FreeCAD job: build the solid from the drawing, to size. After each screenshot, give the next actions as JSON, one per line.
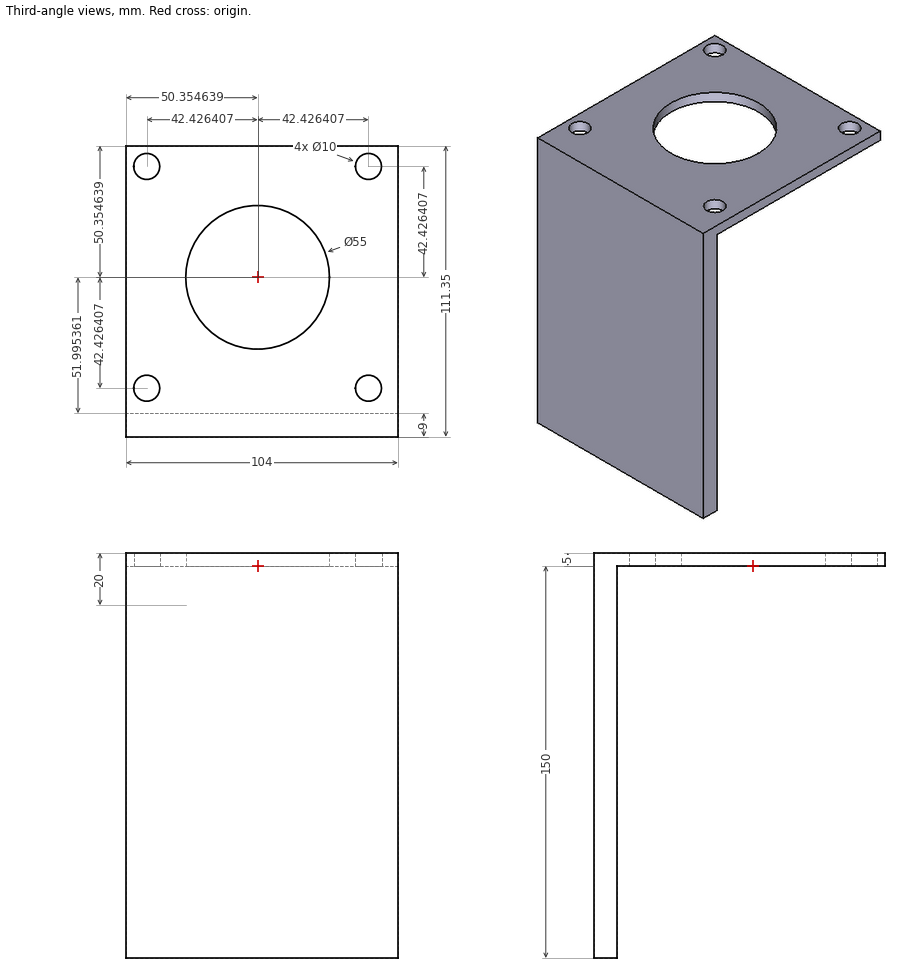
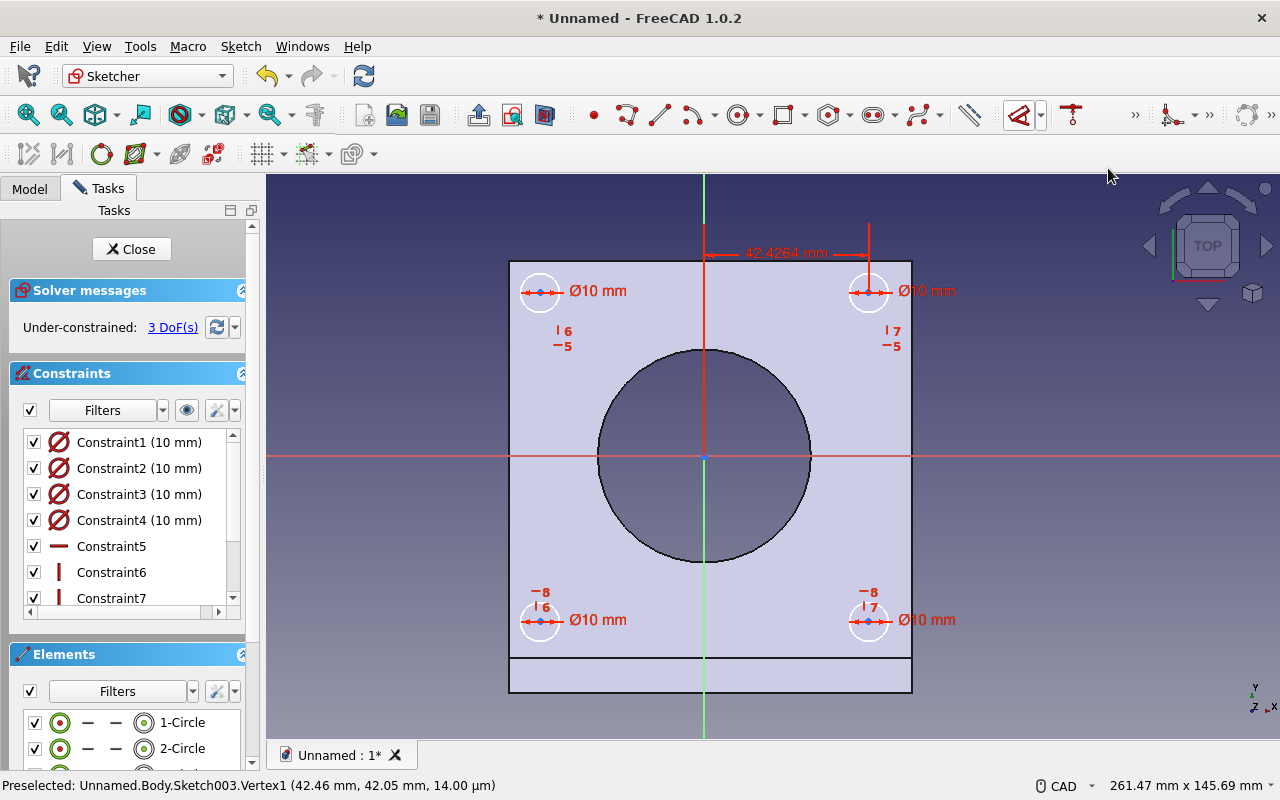
{"action": "left_click", "coordinate": [869, 293]}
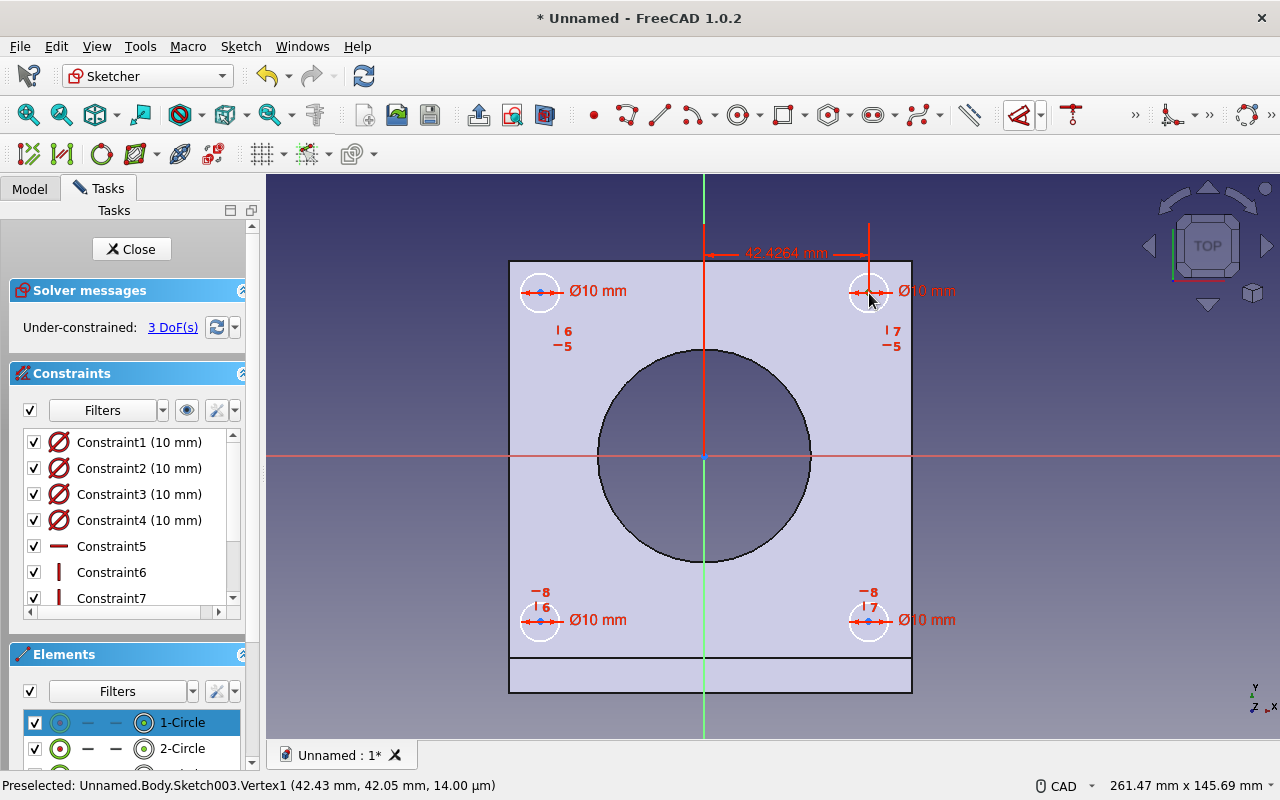
{"action": "left_click", "coordinate": [1040, 116]}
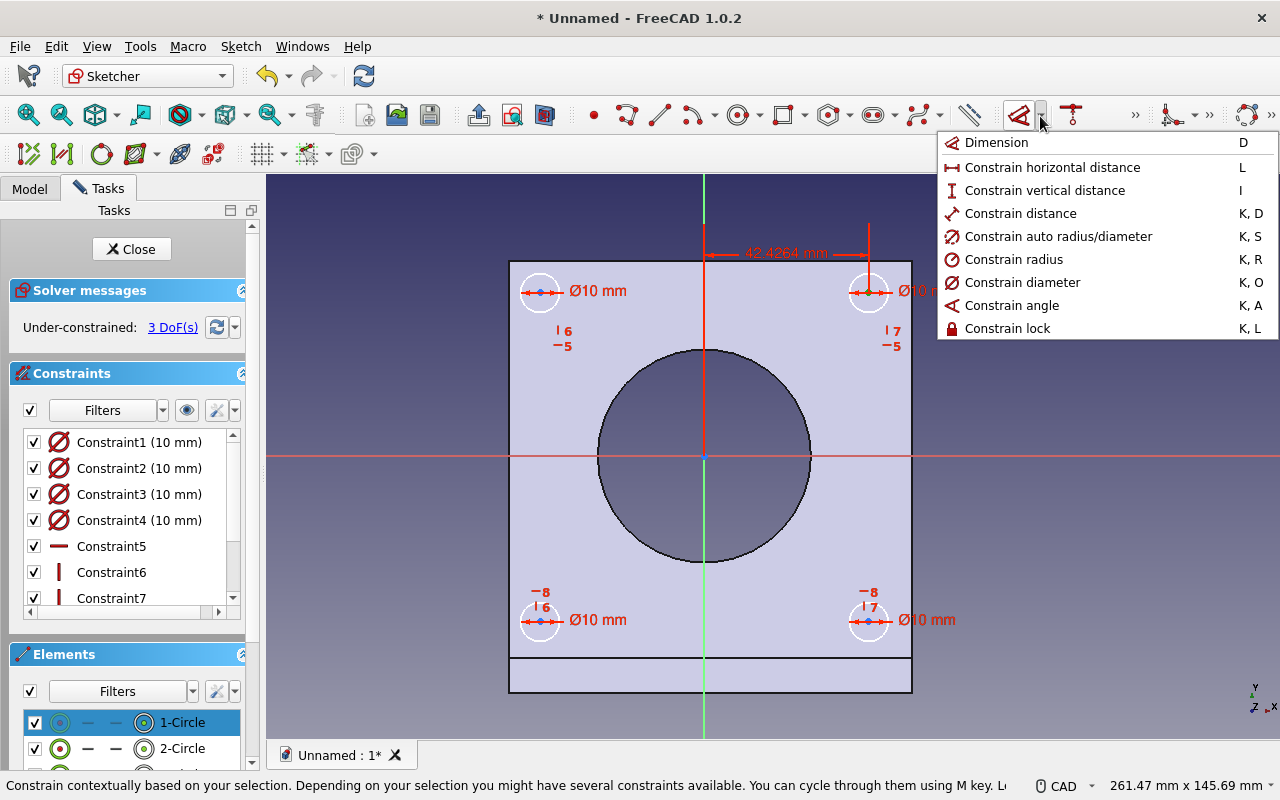
{"action": "left_click", "coordinate": [1108, 190]}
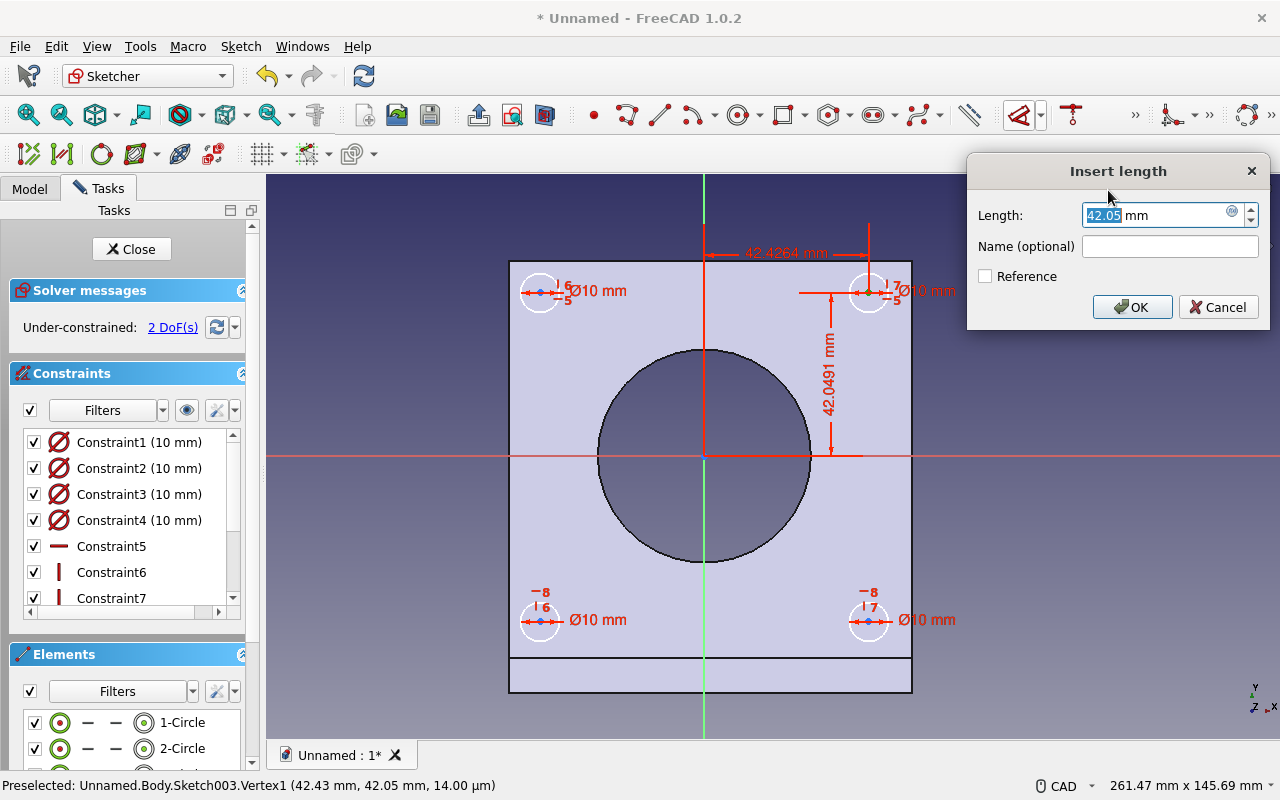
{"action": "type", "text": "42.426407"}
{"action": "key", "text": "Return"}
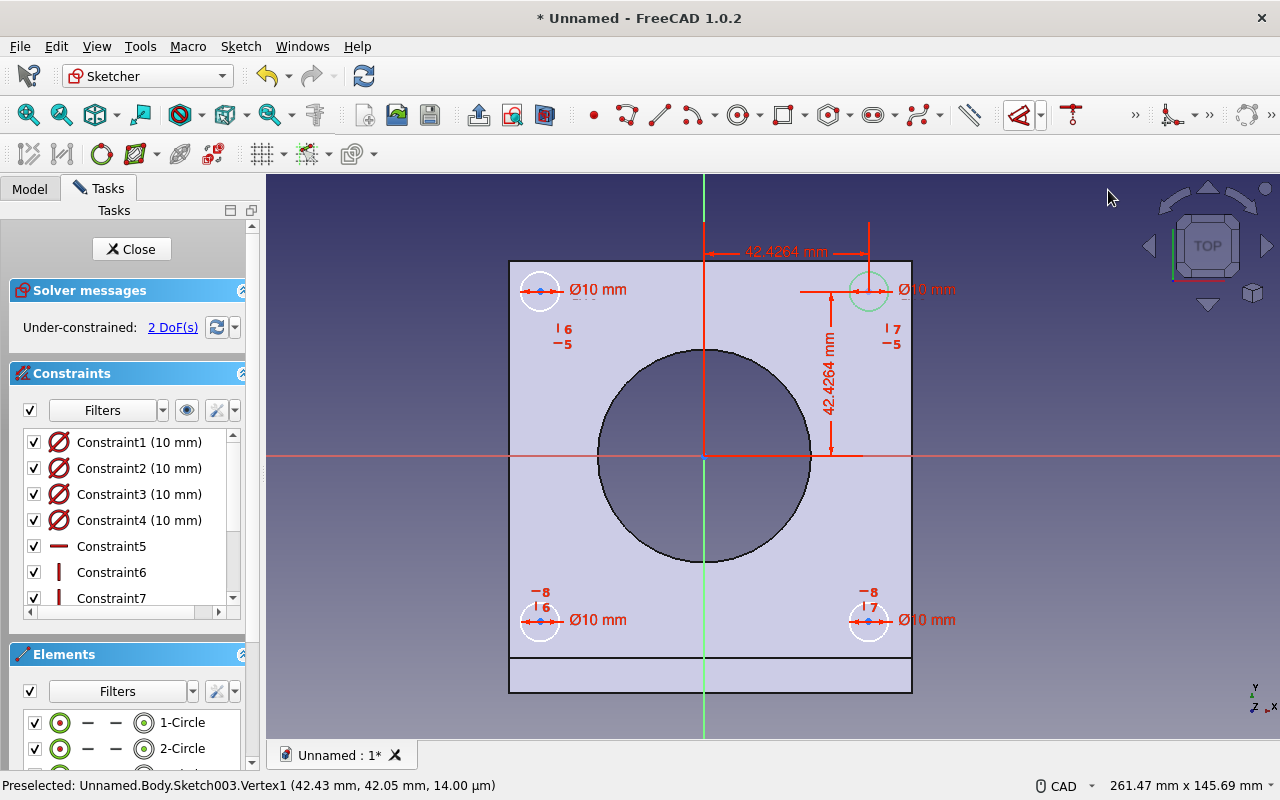
{"action": "left_click", "coordinate": [540, 292]}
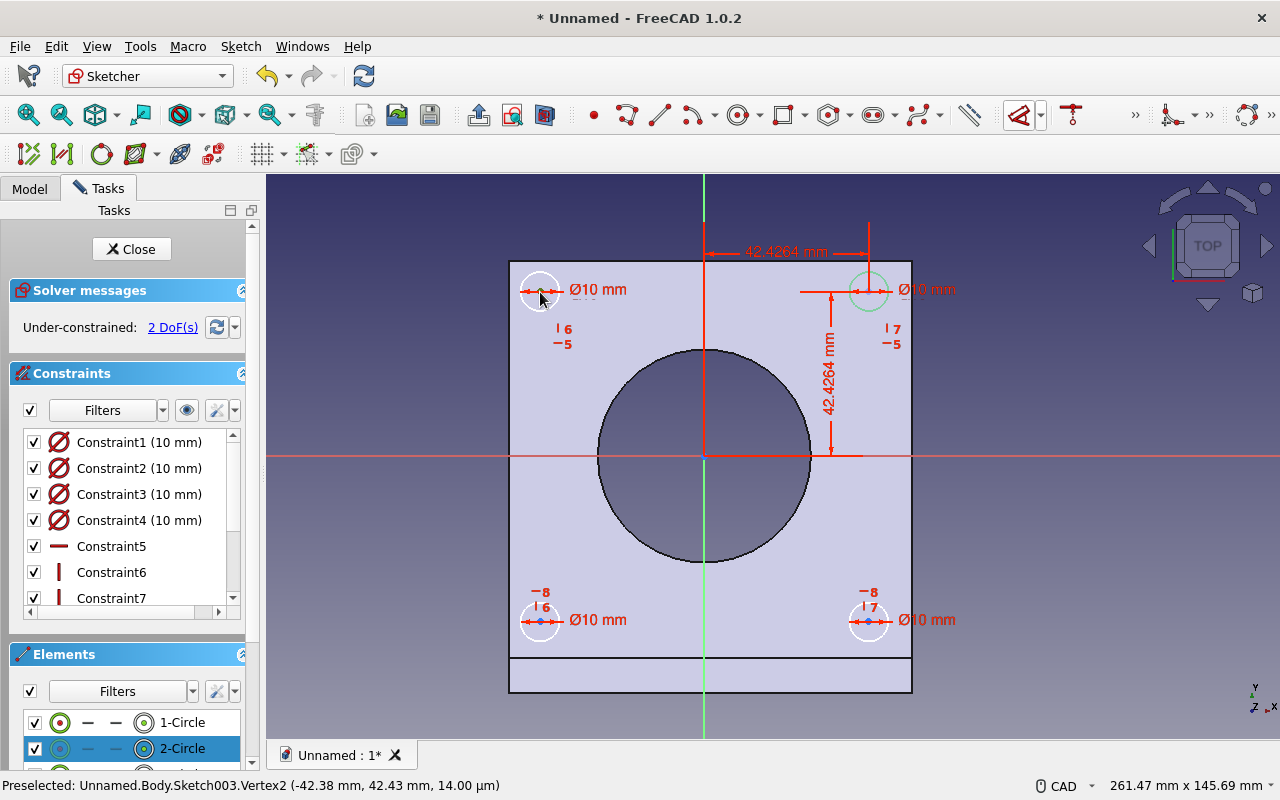
{"action": "key", "text": "l"}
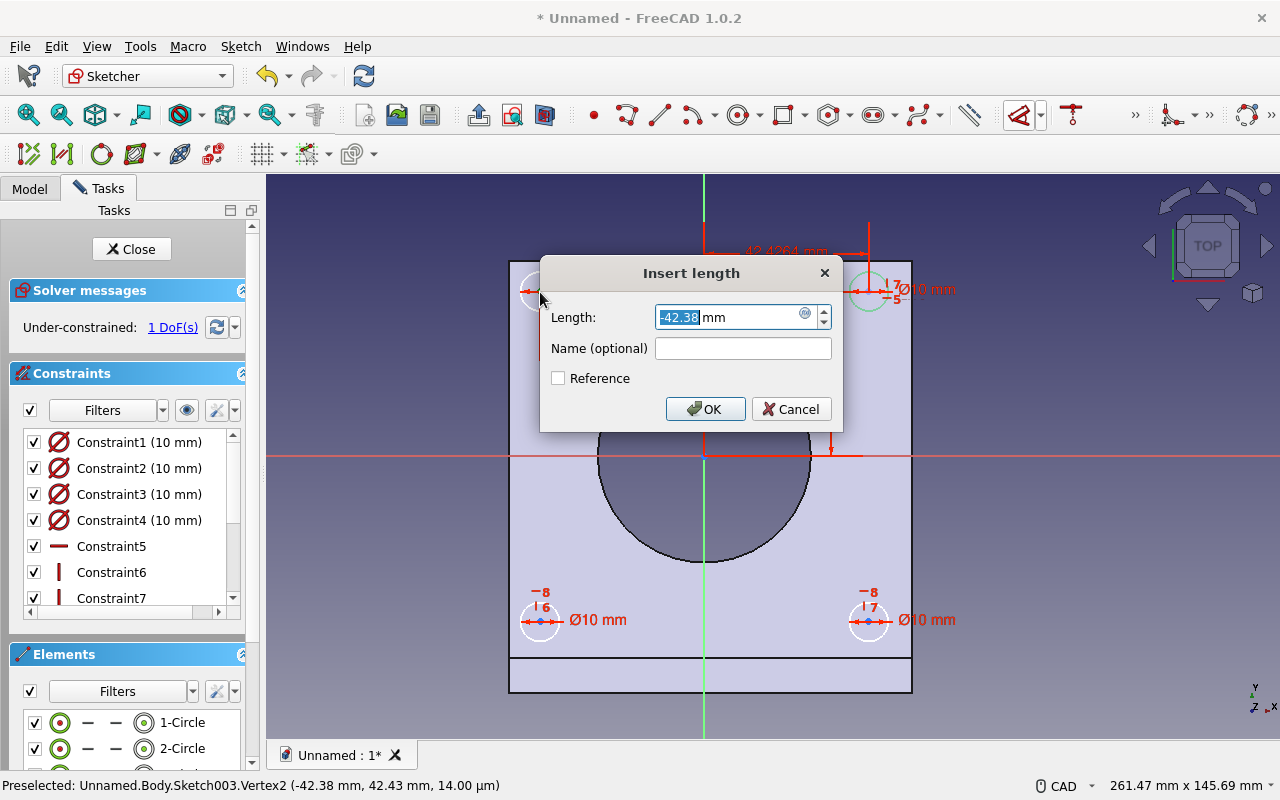
{"action": "type", "text": "-42.426407"}
{"action": "key", "text": "Return"}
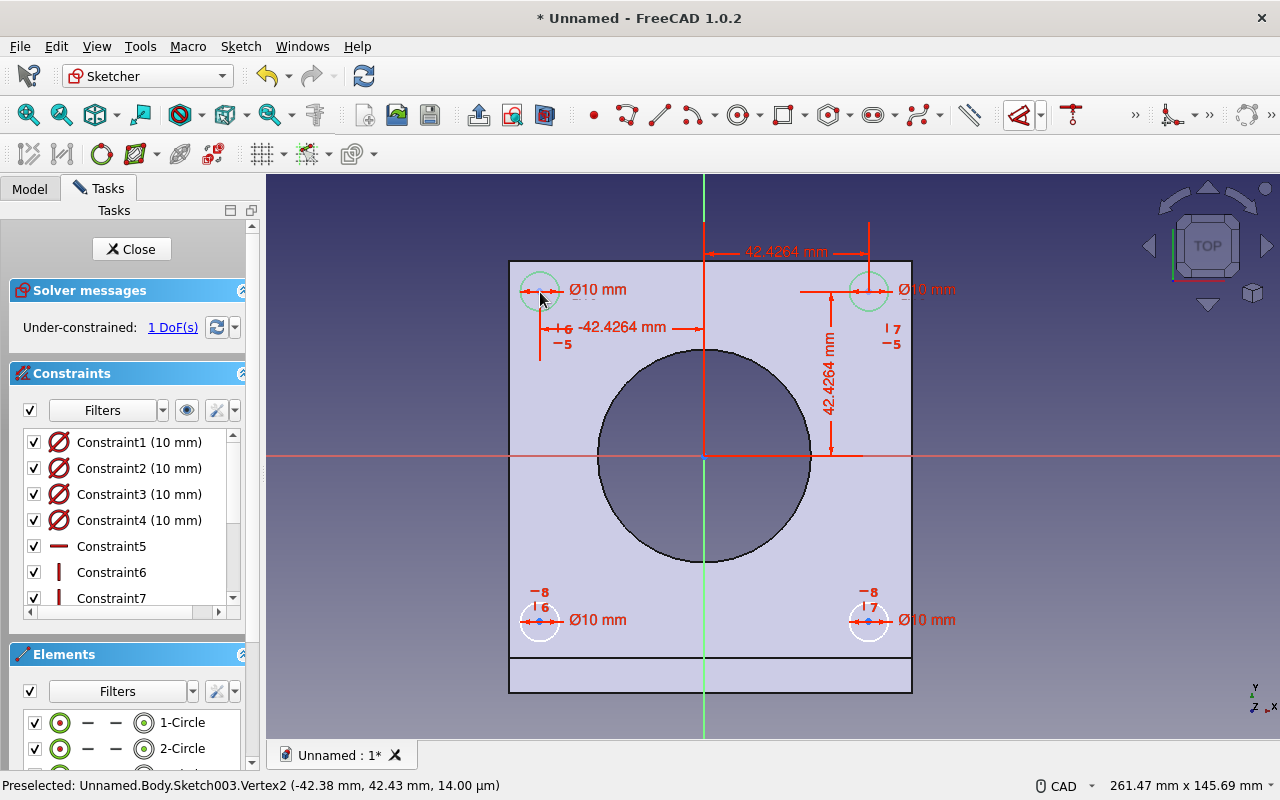
{"action": "left_click", "coordinate": [540, 622]}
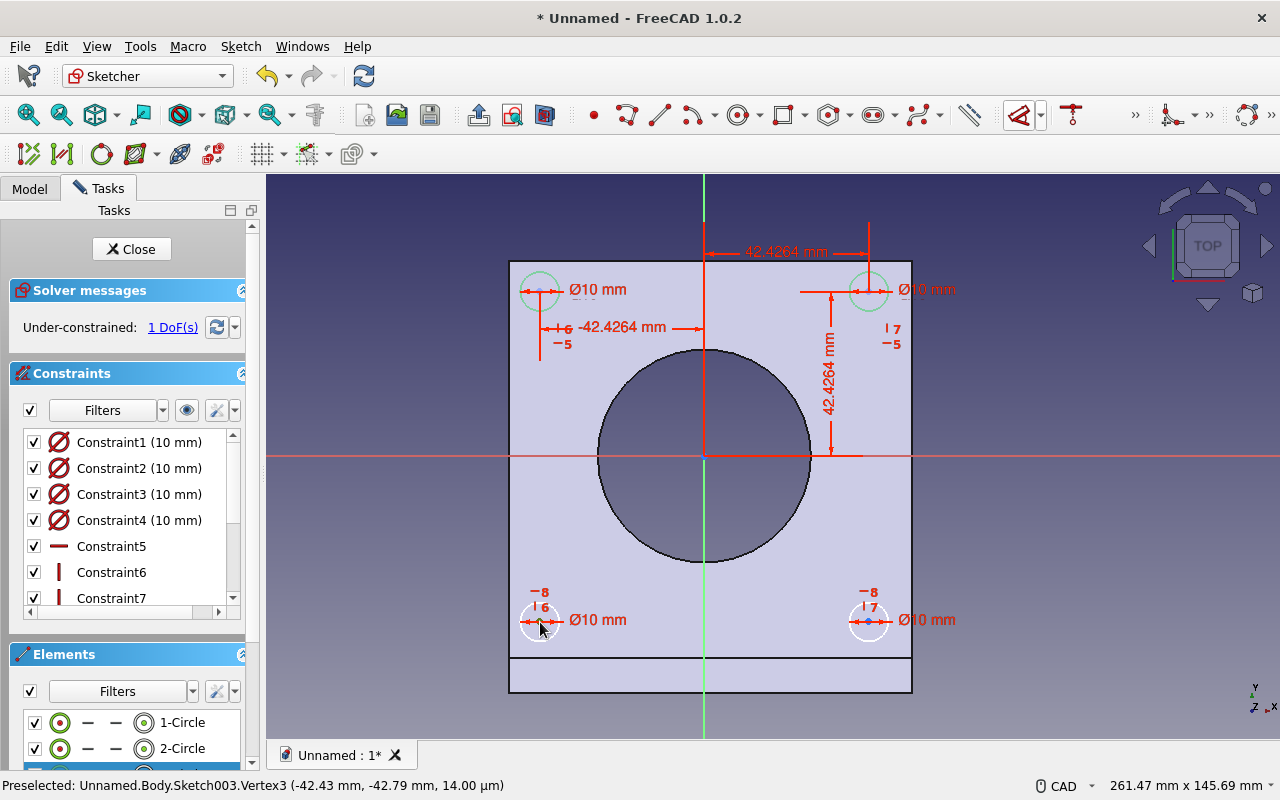
{"action": "left_click", "coordinate": [1040, 116]}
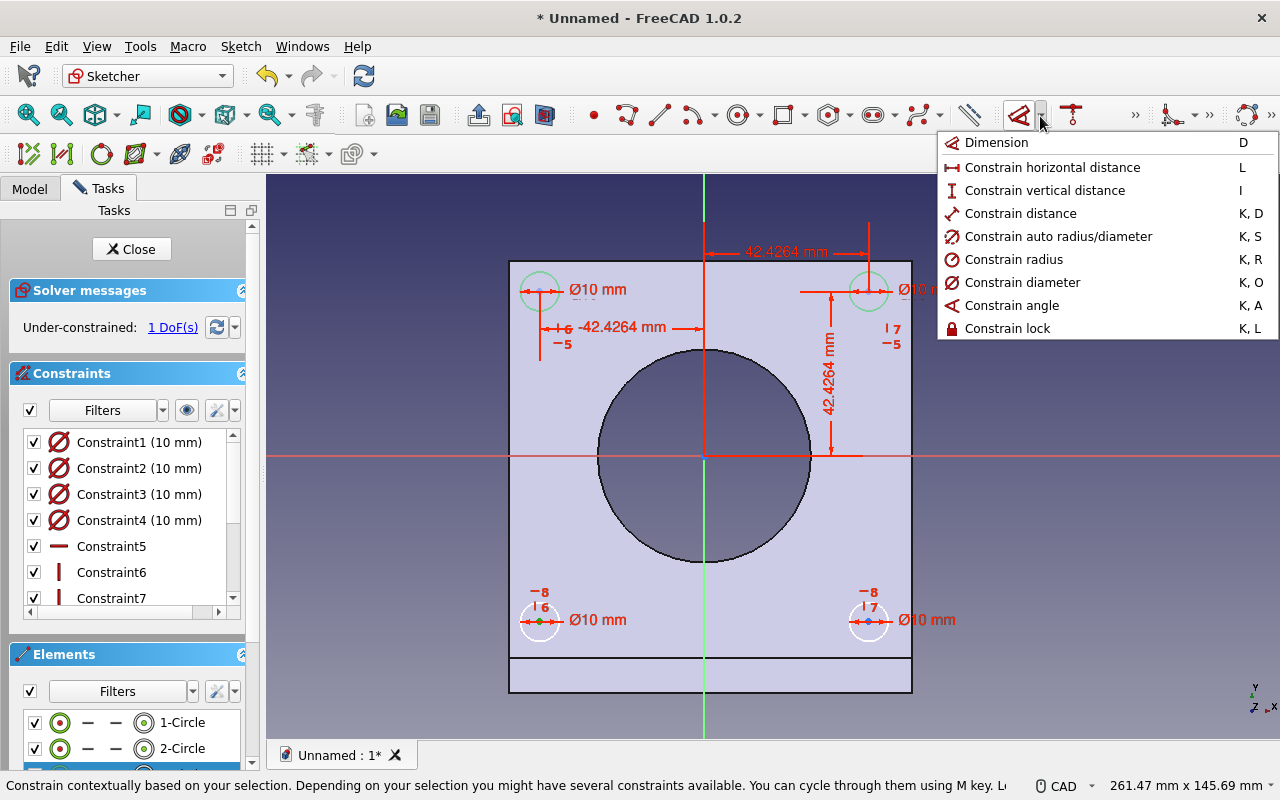
{"action": "left_click", "coordinate": [1108, 190]}